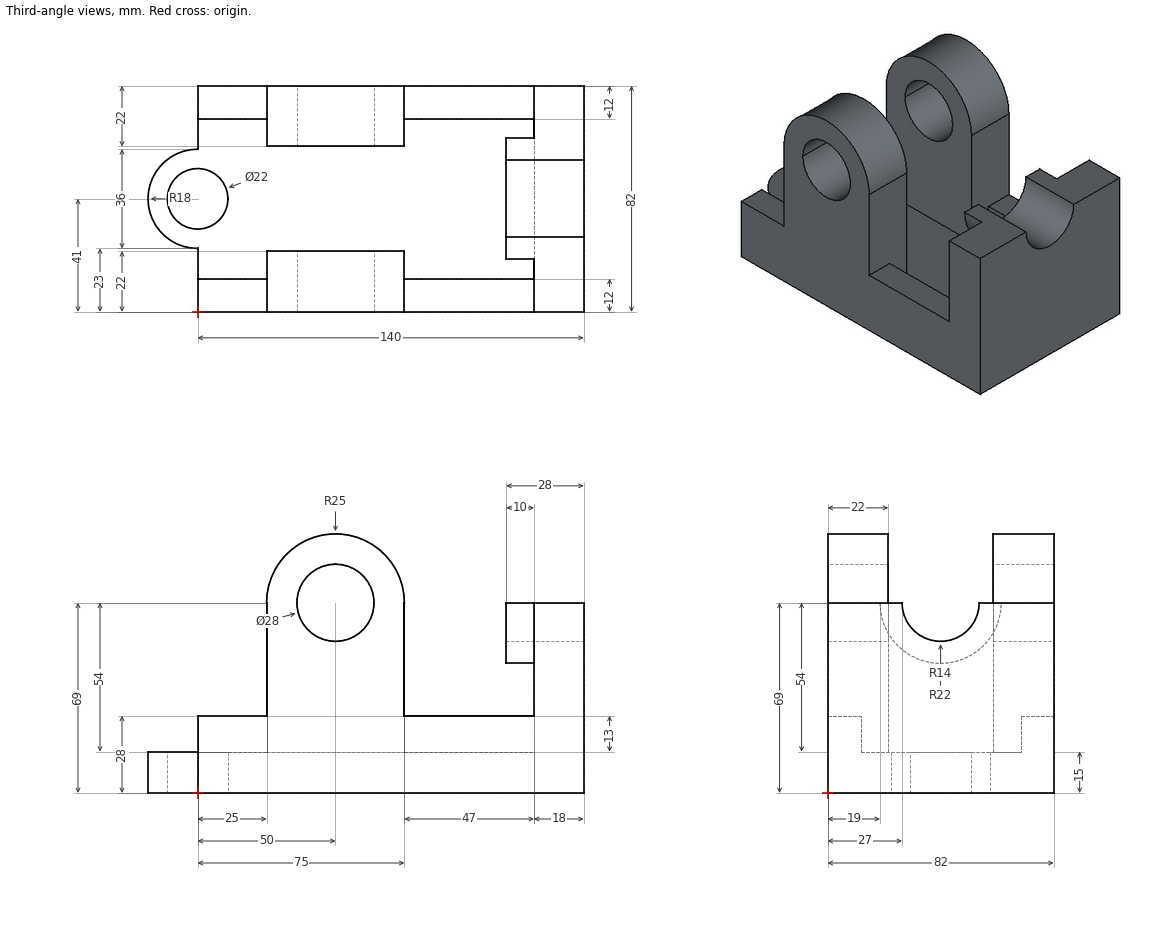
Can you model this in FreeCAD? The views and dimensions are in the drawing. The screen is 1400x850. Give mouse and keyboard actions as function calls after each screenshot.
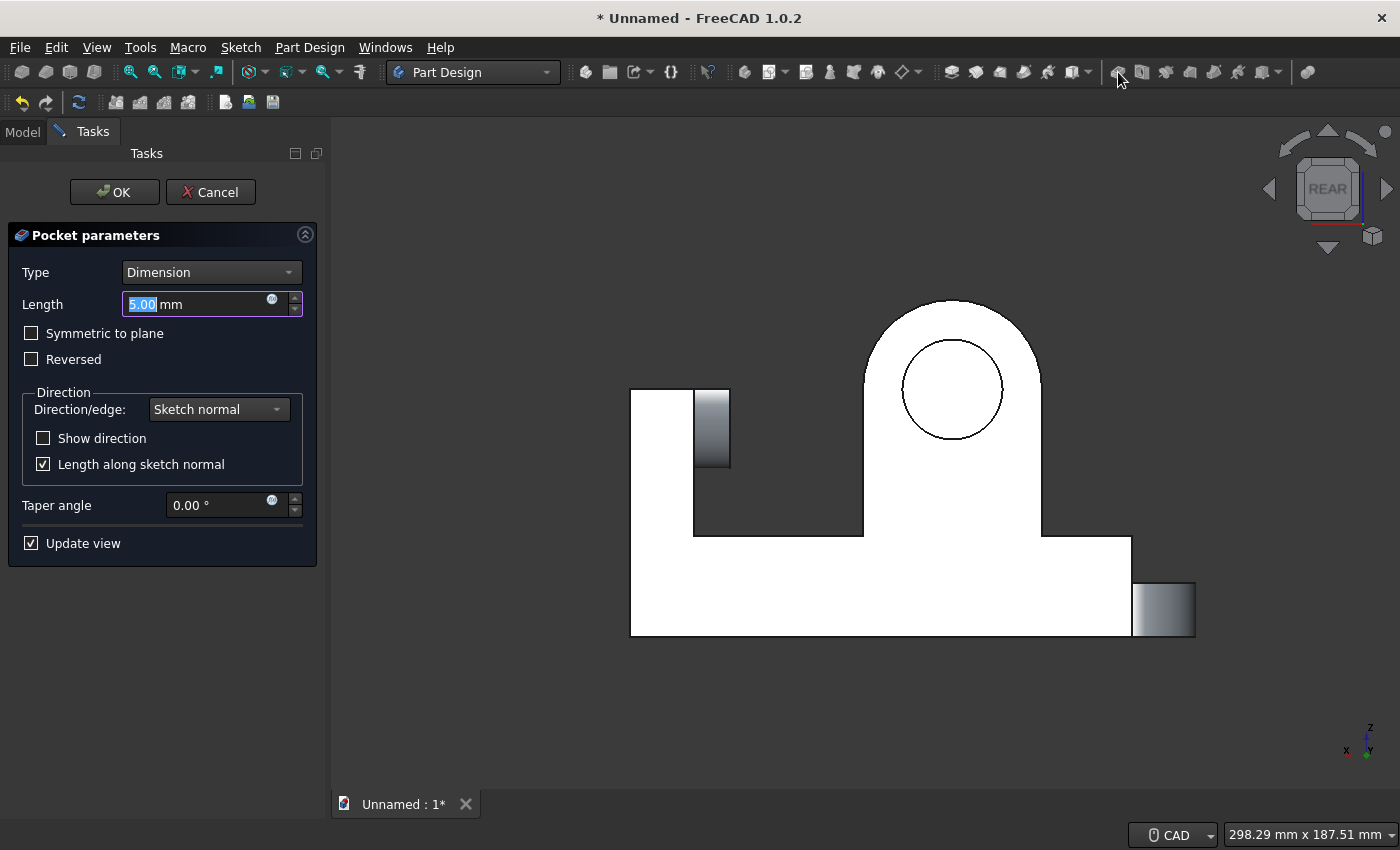
text(22)
key(Tab)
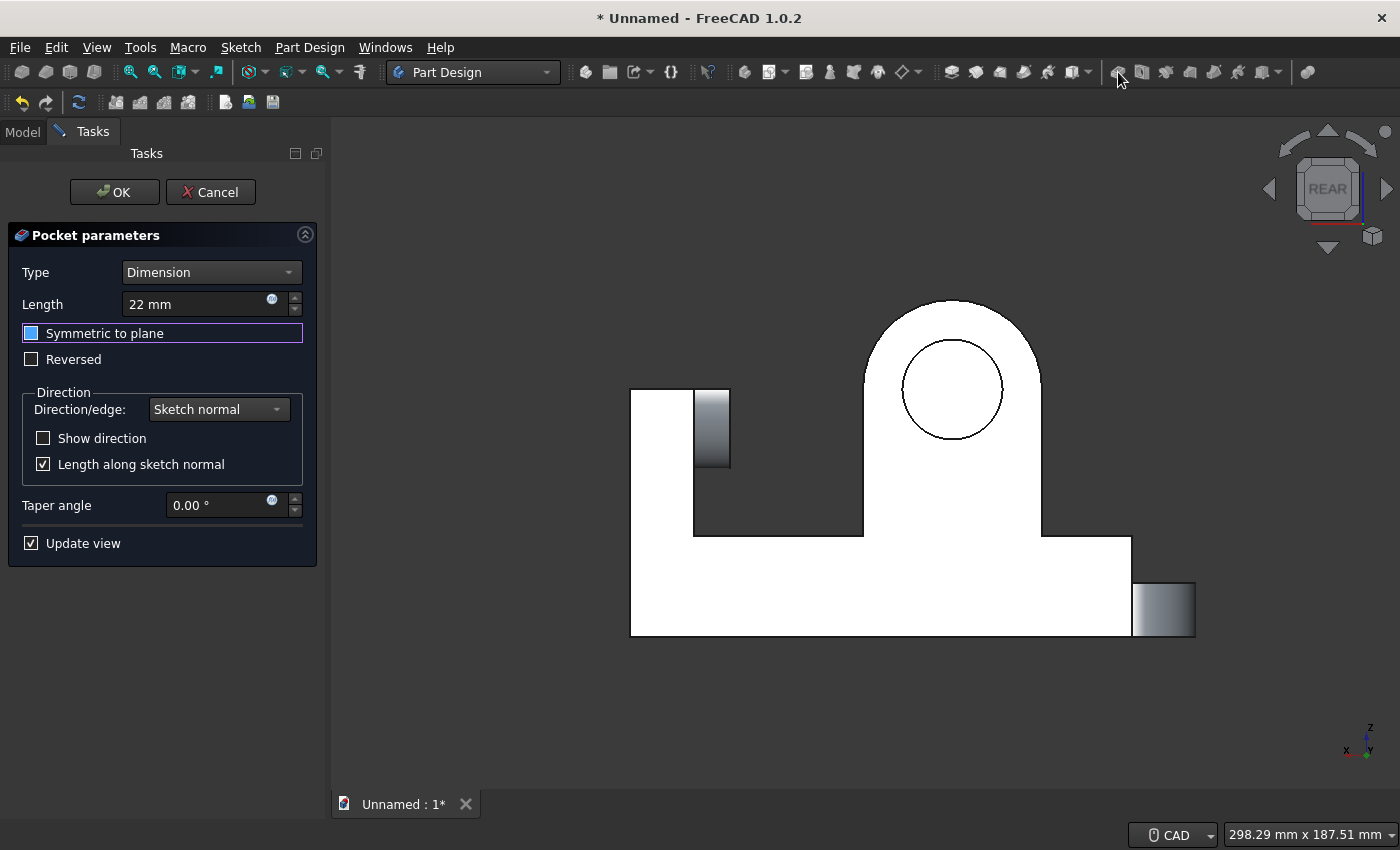
click(115, 192)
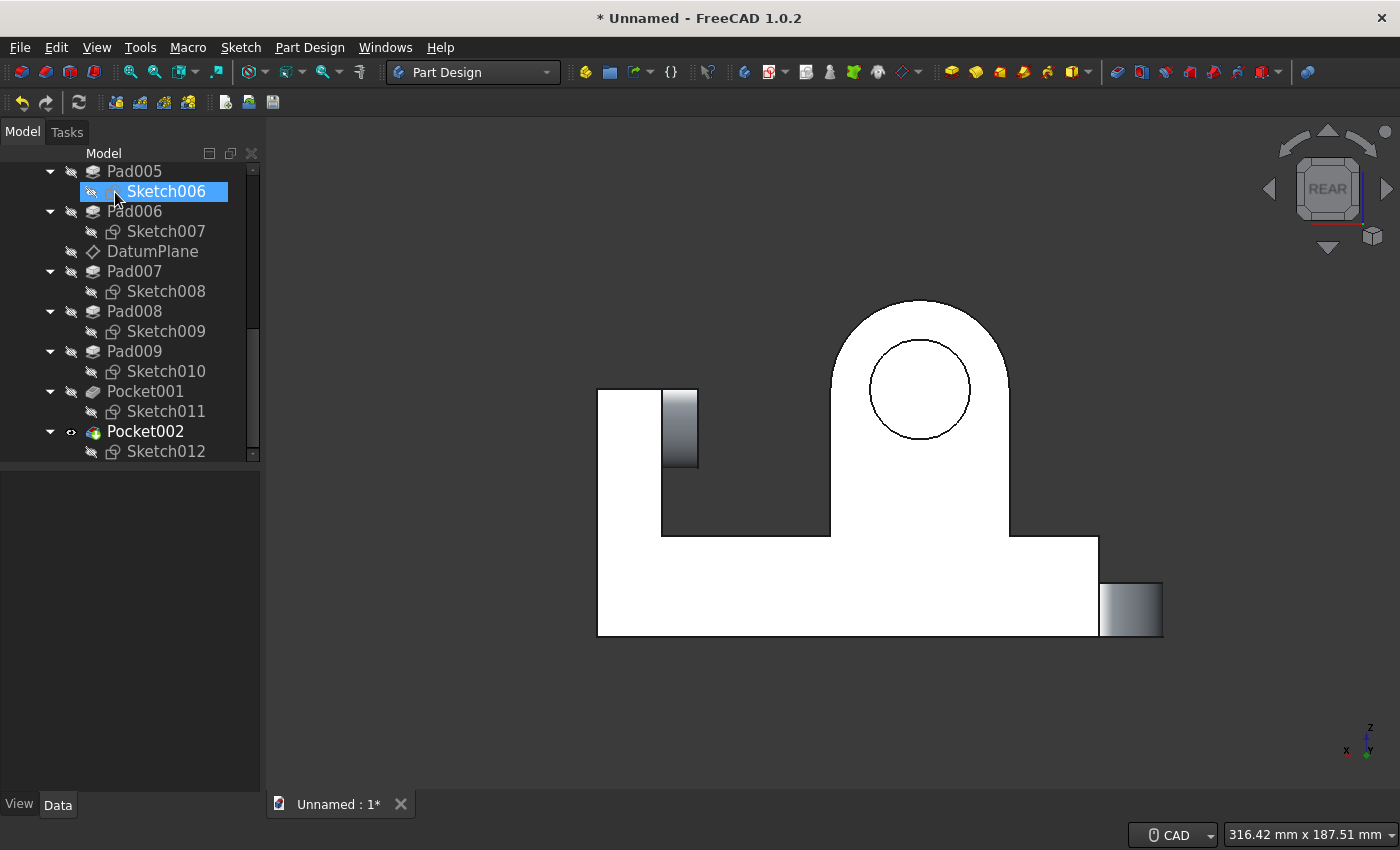
click(920, 400)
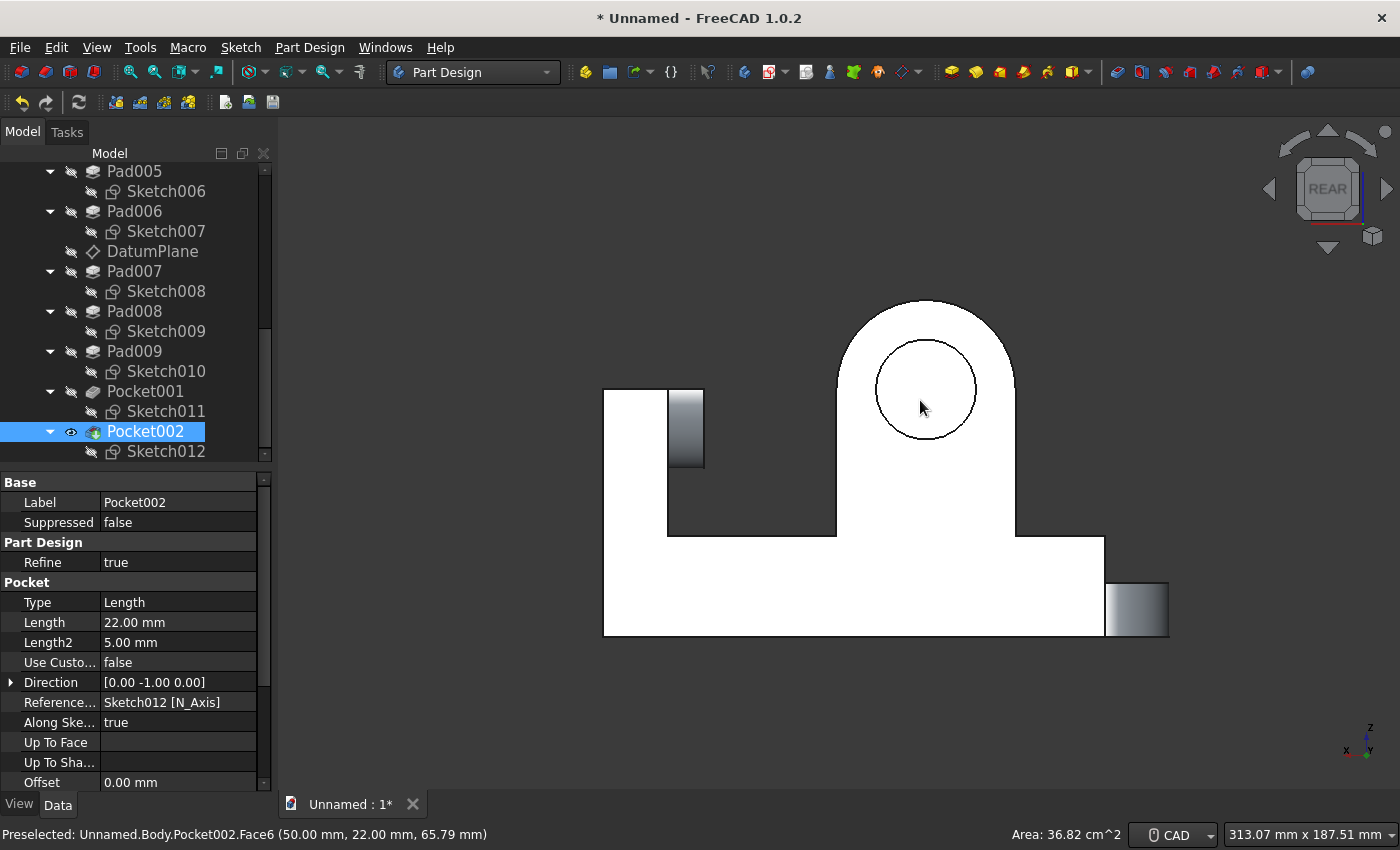
click(770, 72)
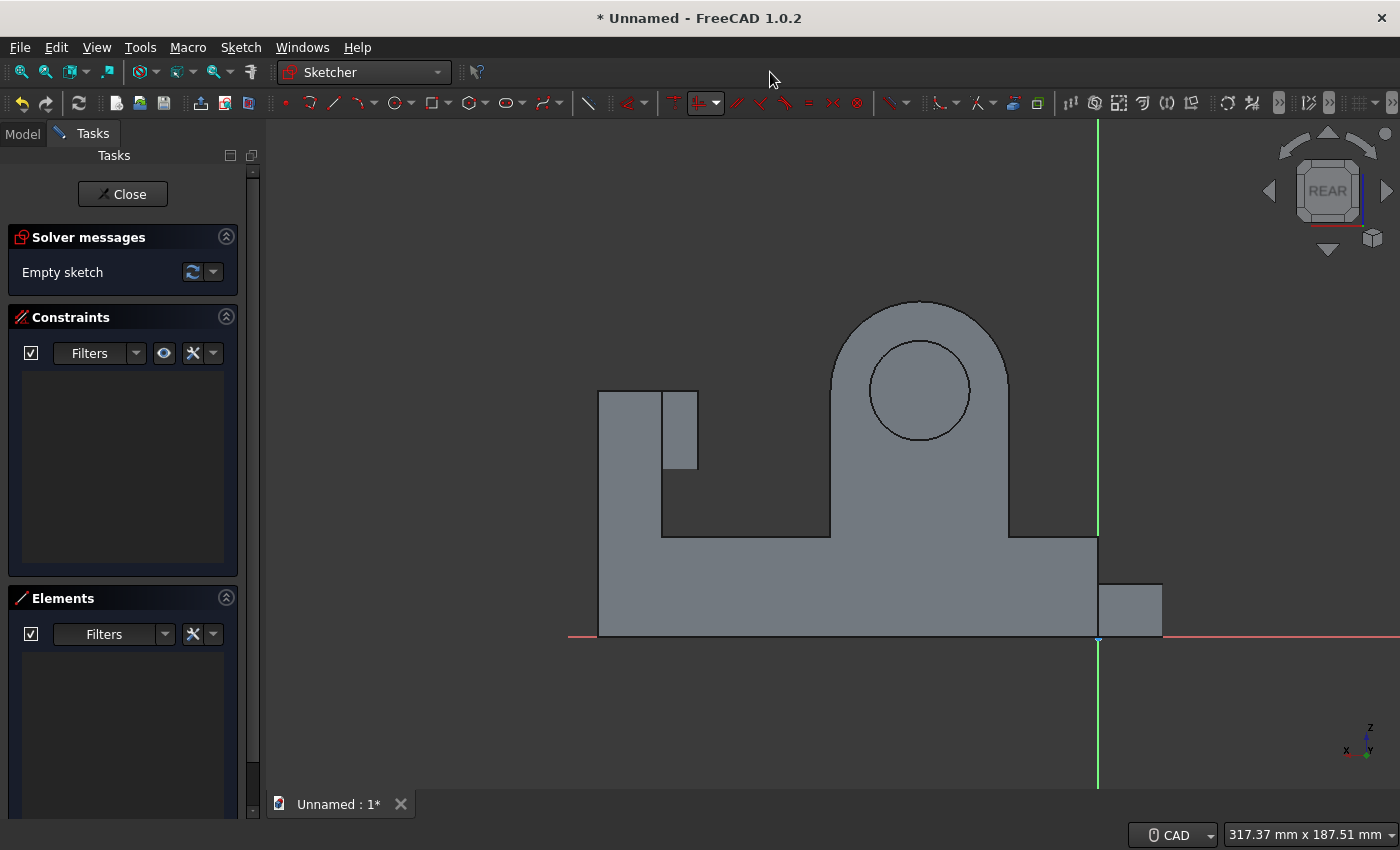
scroll(971, 370, up, 7)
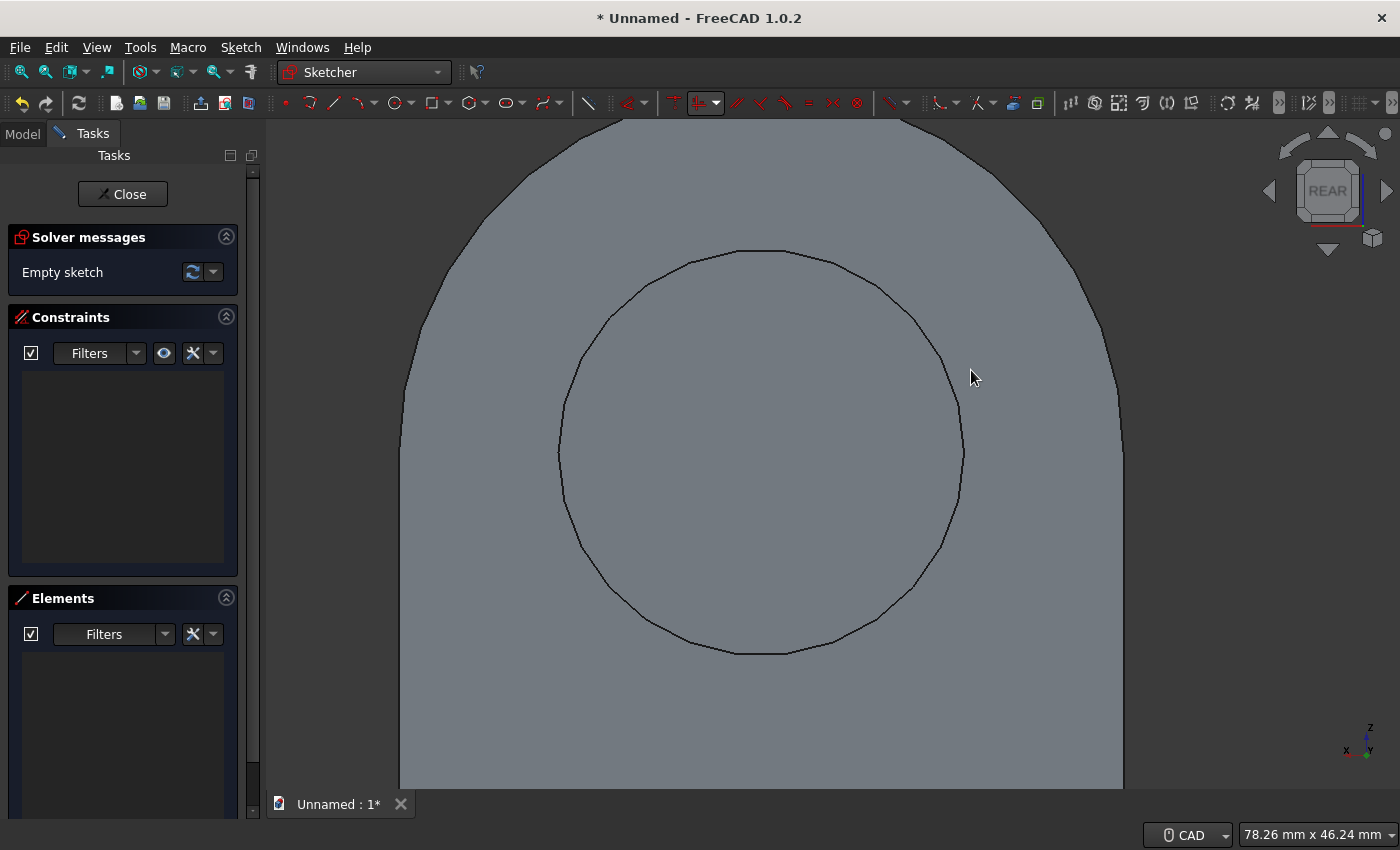
click(396, 104)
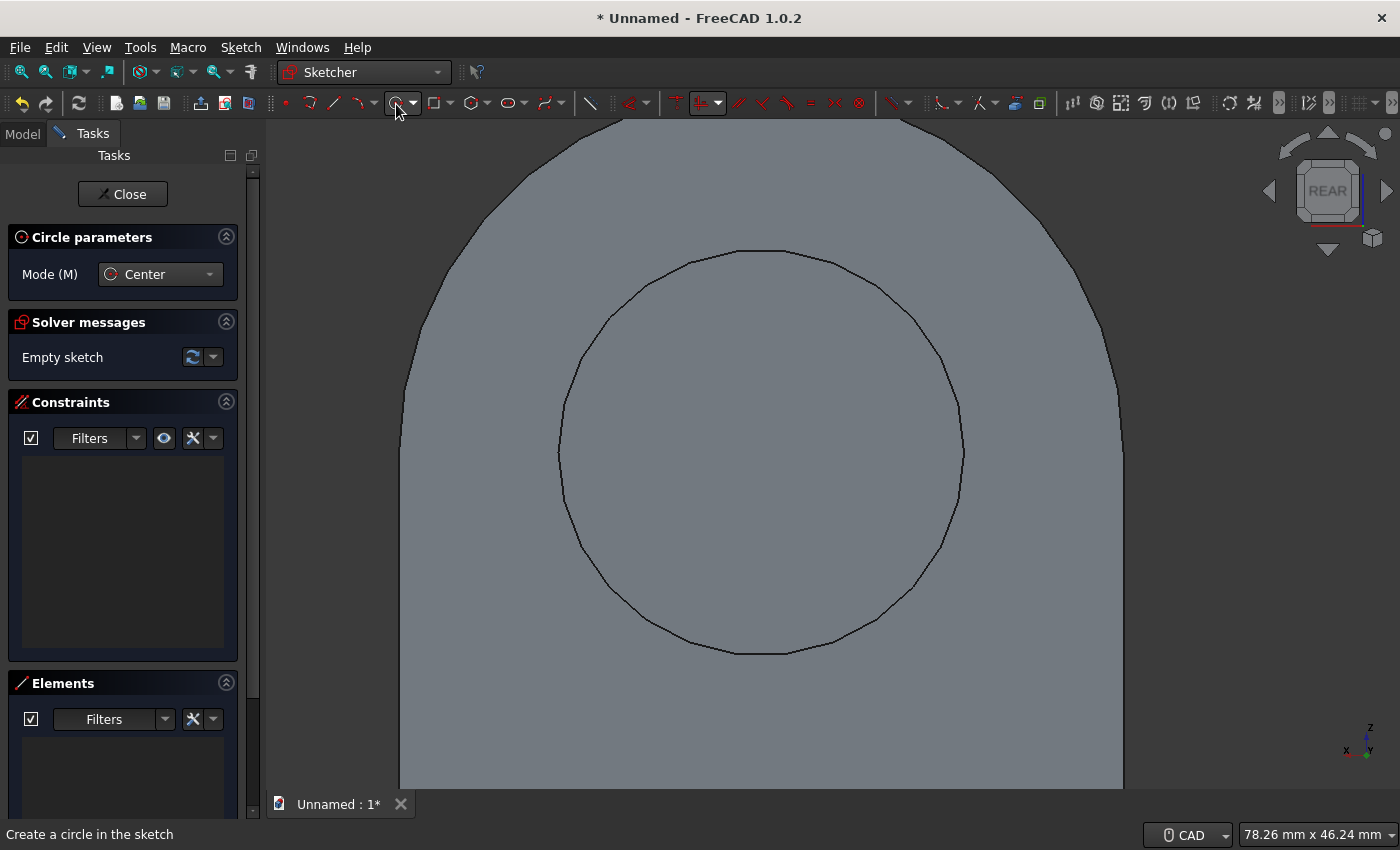
click(761, 453)
click(905, 309)
key(Escape)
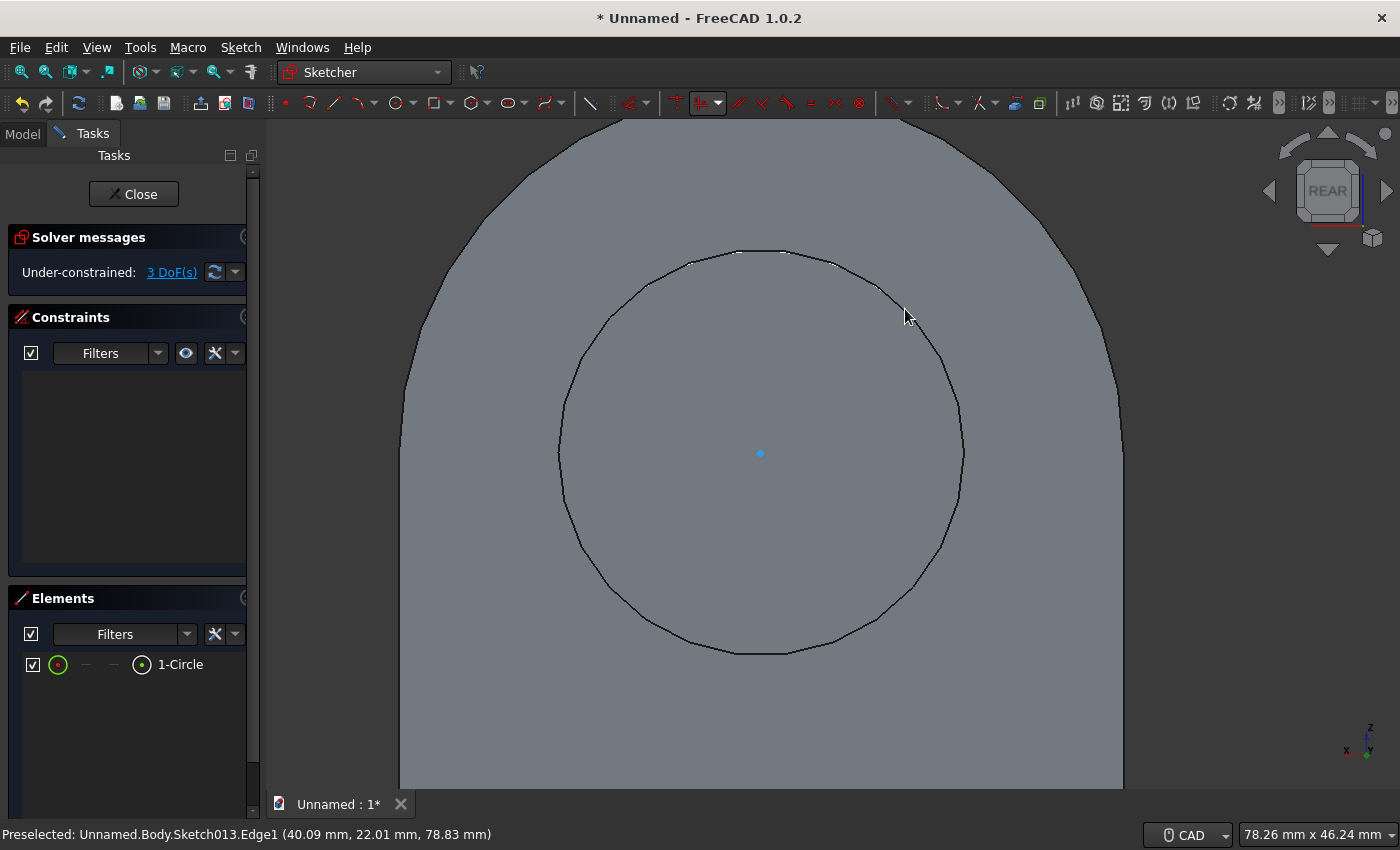
click(630, 104)